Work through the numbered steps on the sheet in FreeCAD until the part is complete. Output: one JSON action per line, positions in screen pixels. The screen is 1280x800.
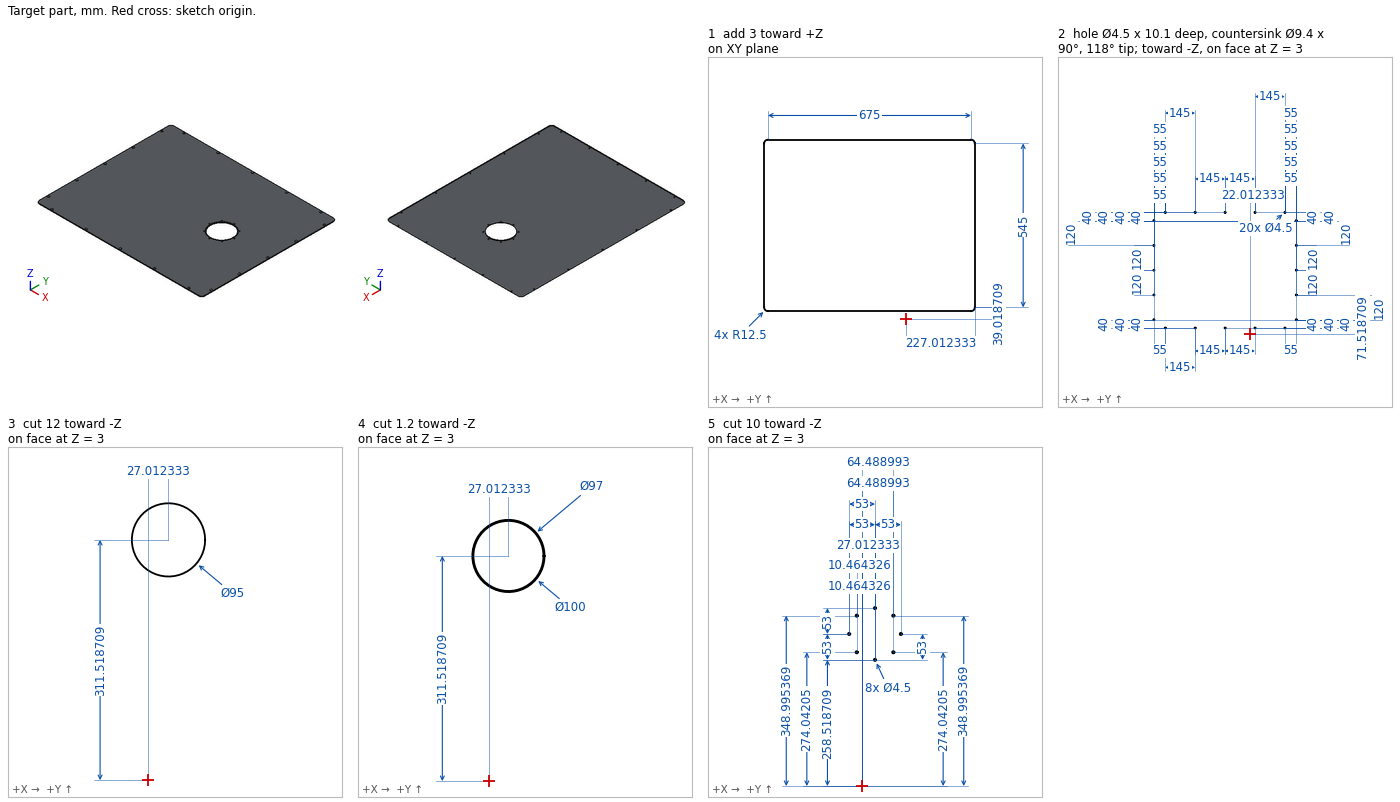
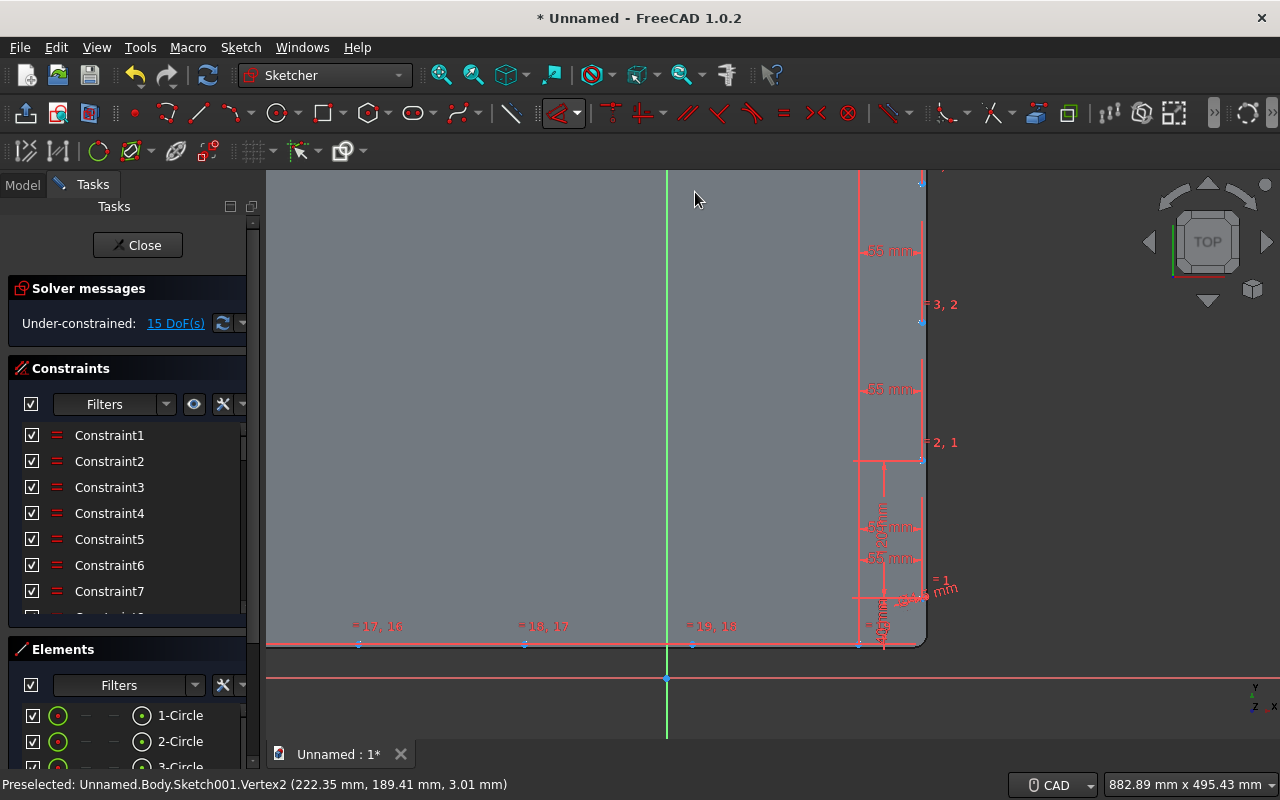
{"action": "left_click", "coordinate": [922, 461]}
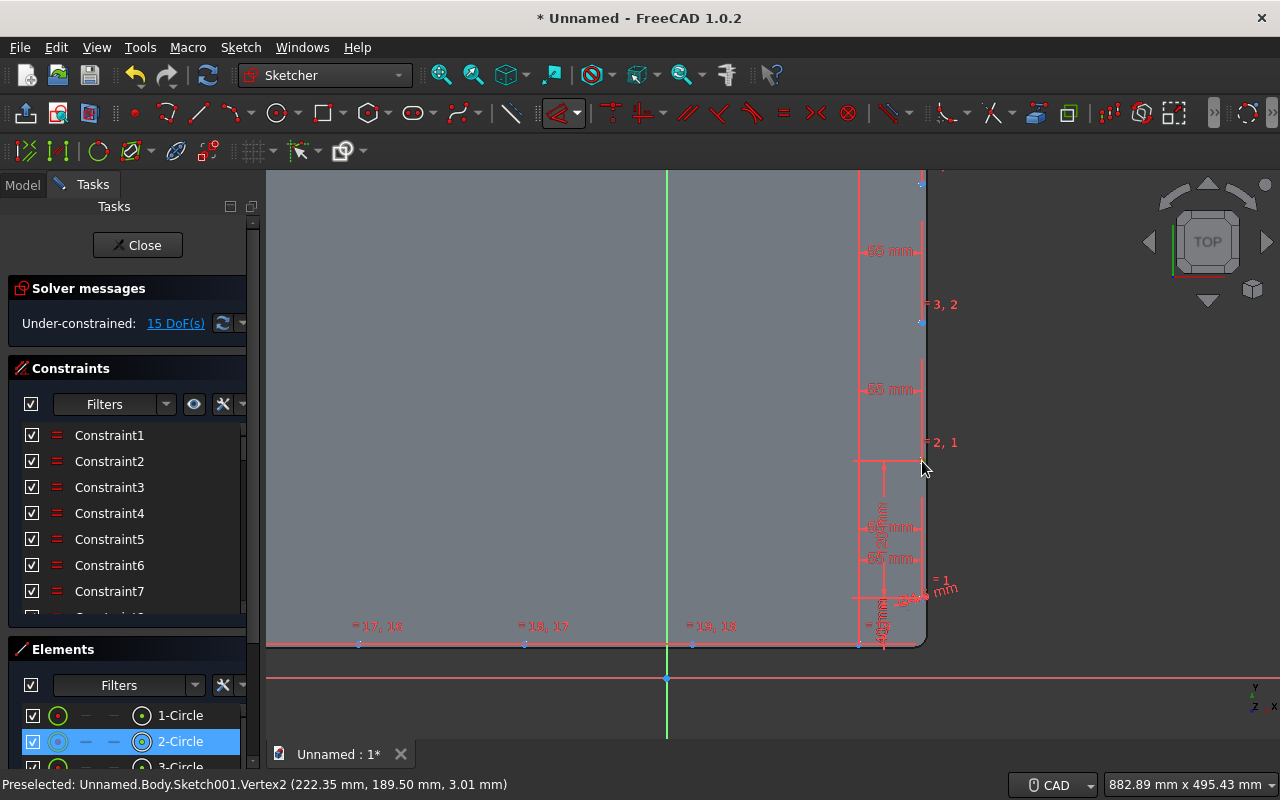
{"action": "left_click", "coordinate": [922, 322]}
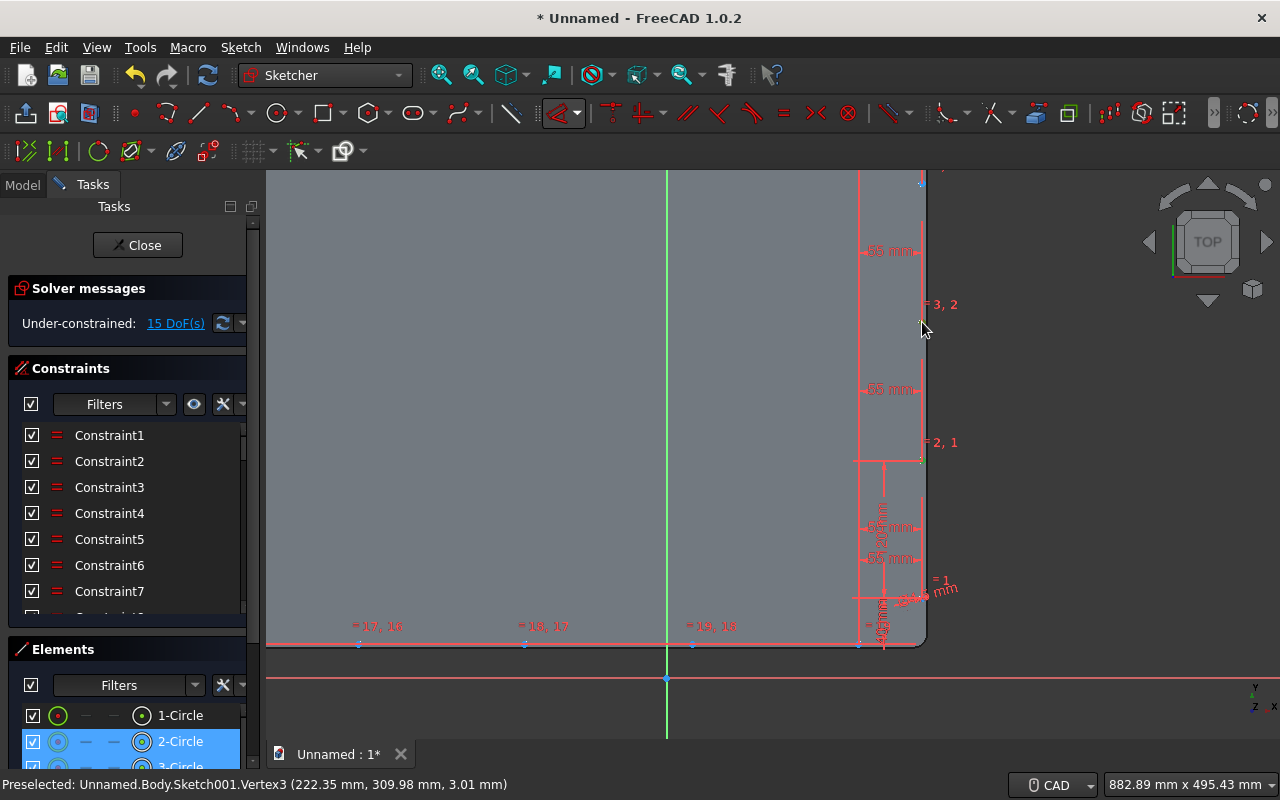
{"action": "left_click", "coordinate": [580, 114]}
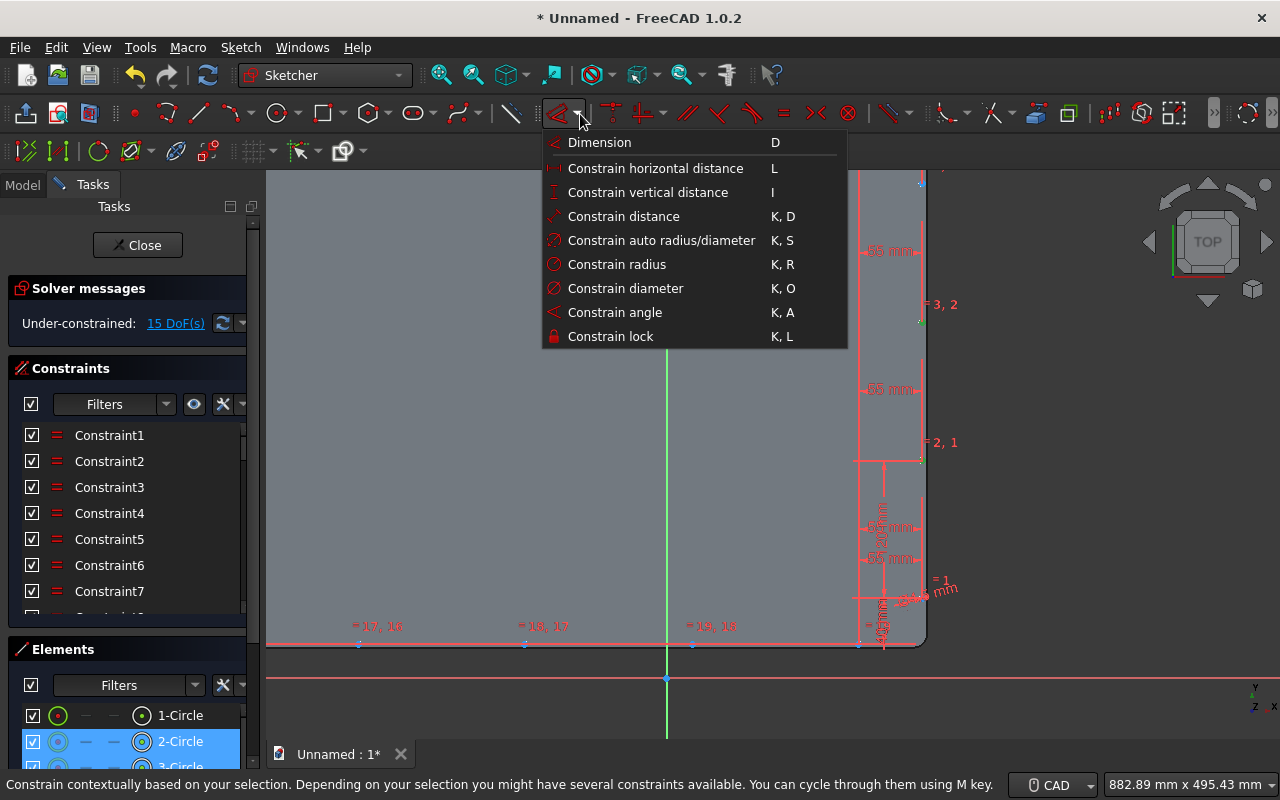
{"action": "left_click", "coordinate": [695, 192]}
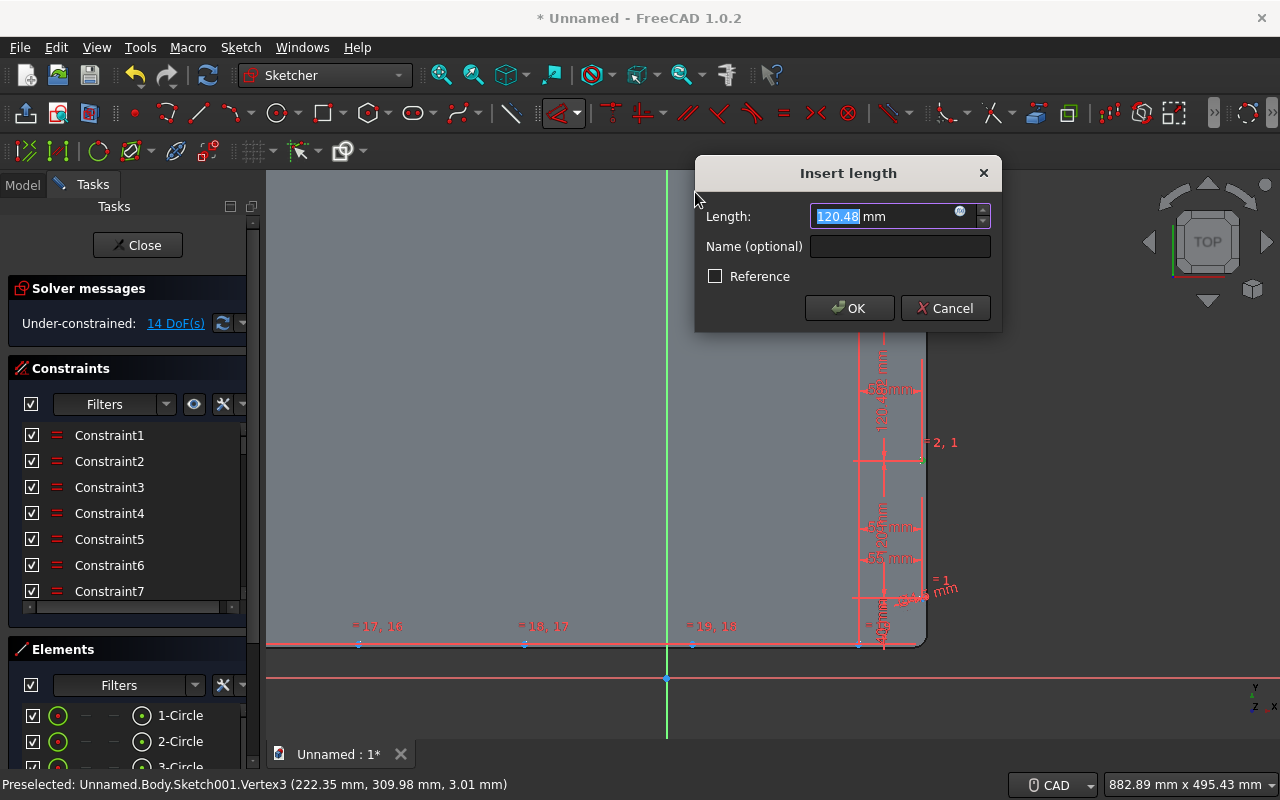
{"action": "type", "text": "120"}
{"action": "key", "text": "Return"}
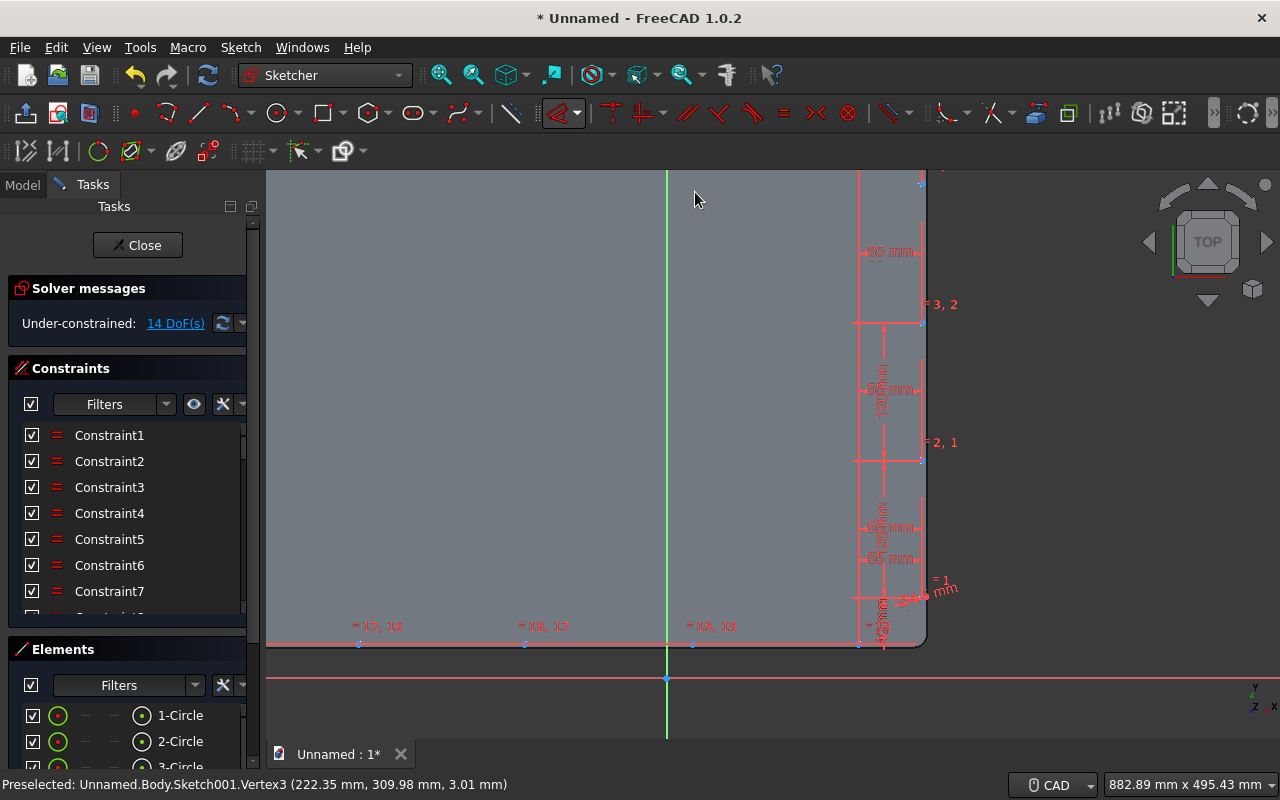
{"action": "left_click", "coordinate": [922, 323]}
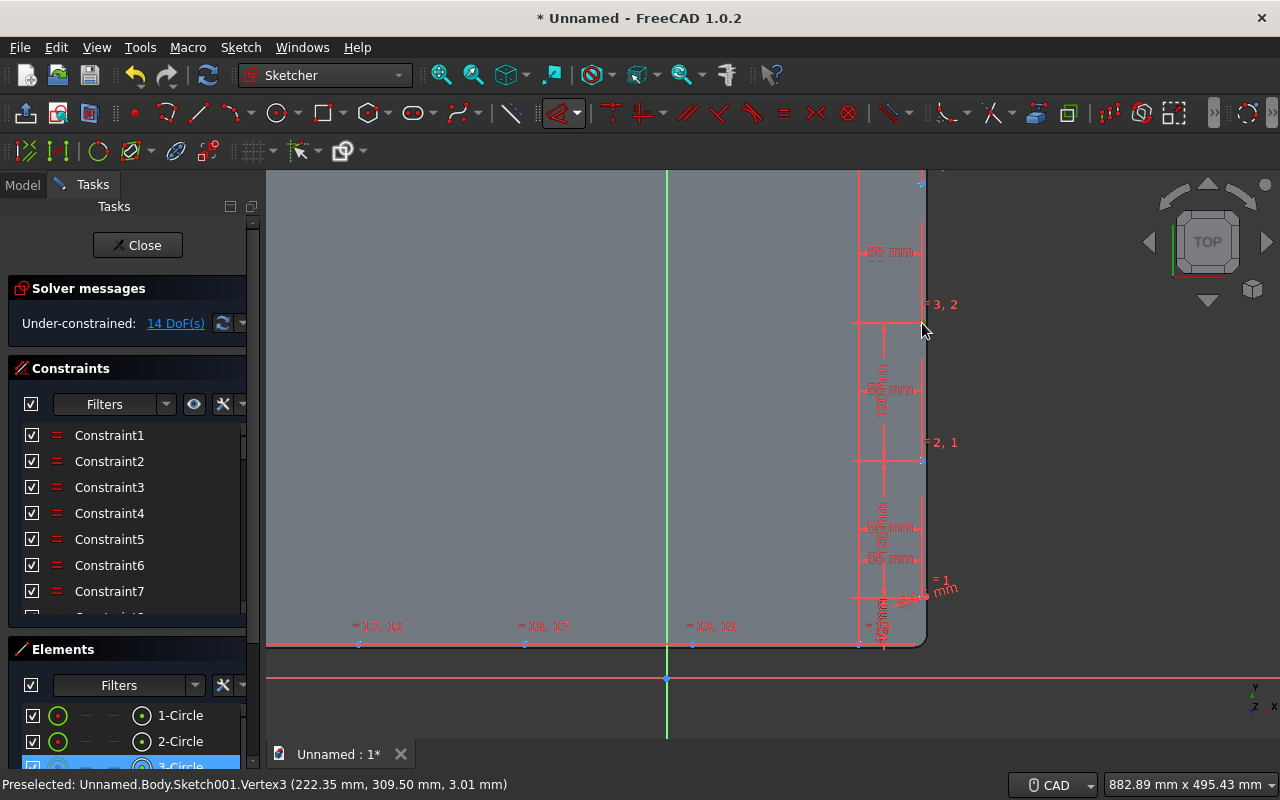
{"action": "scroll", "coordinate": [922, 597], "scroll_direction": "down", "scroll_amount": 3}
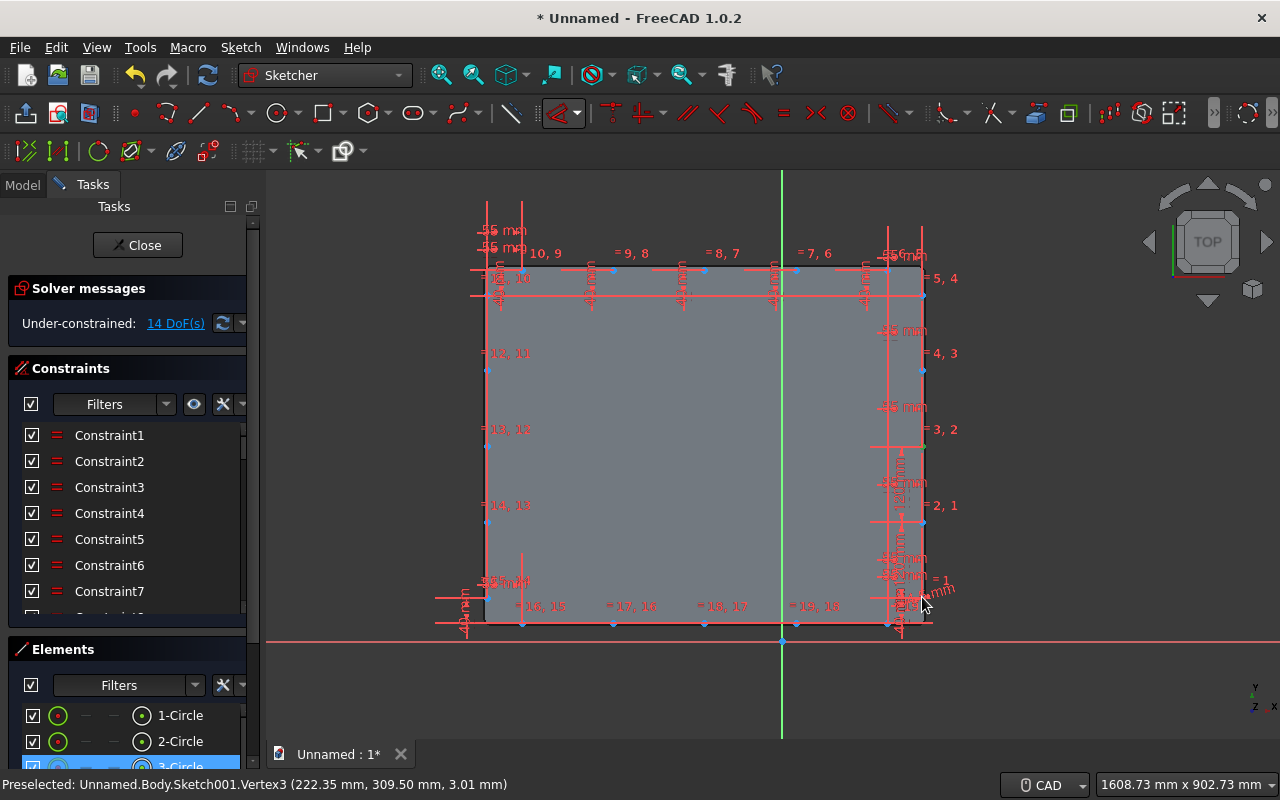
{"action": "left_click", "coordinate": [922, 370]}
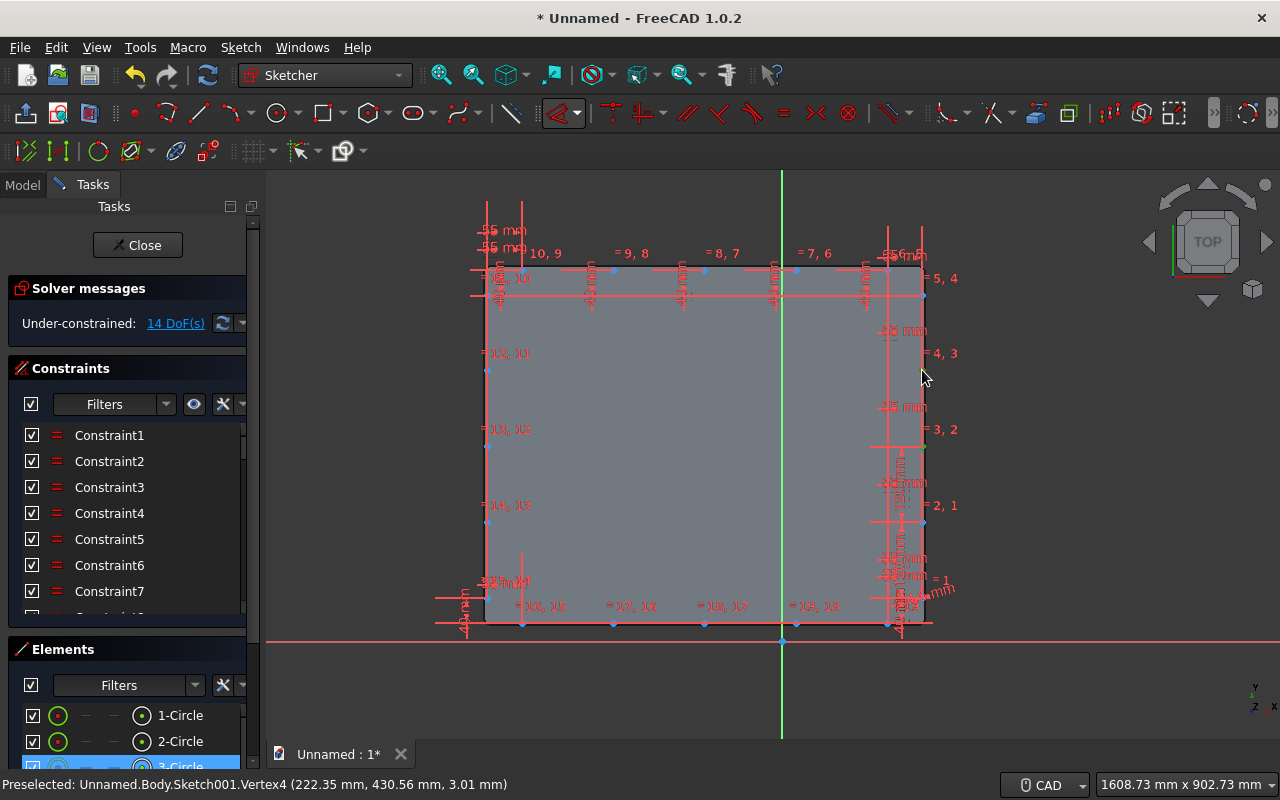
{"action": "left_click", "coordinate": [580, 114]}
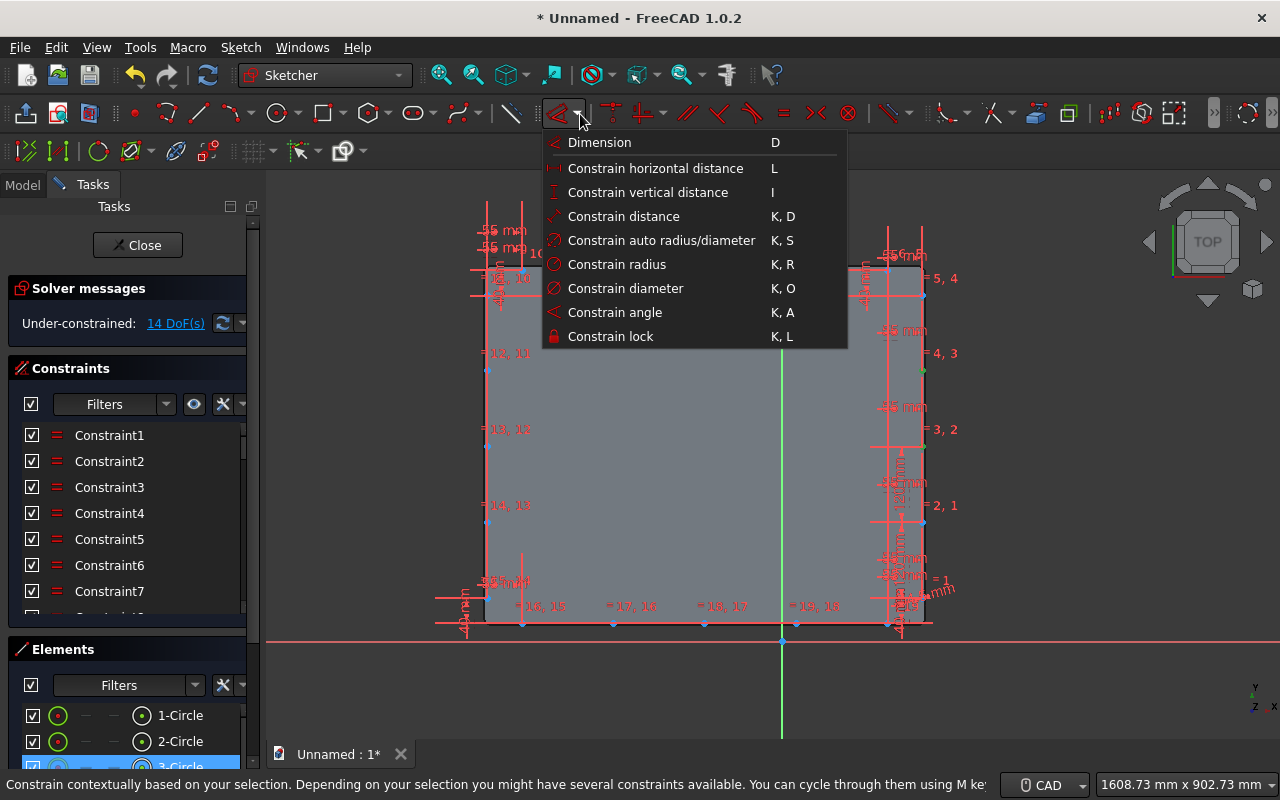
{"action": "left_click", "coordinate": [695, 192]}